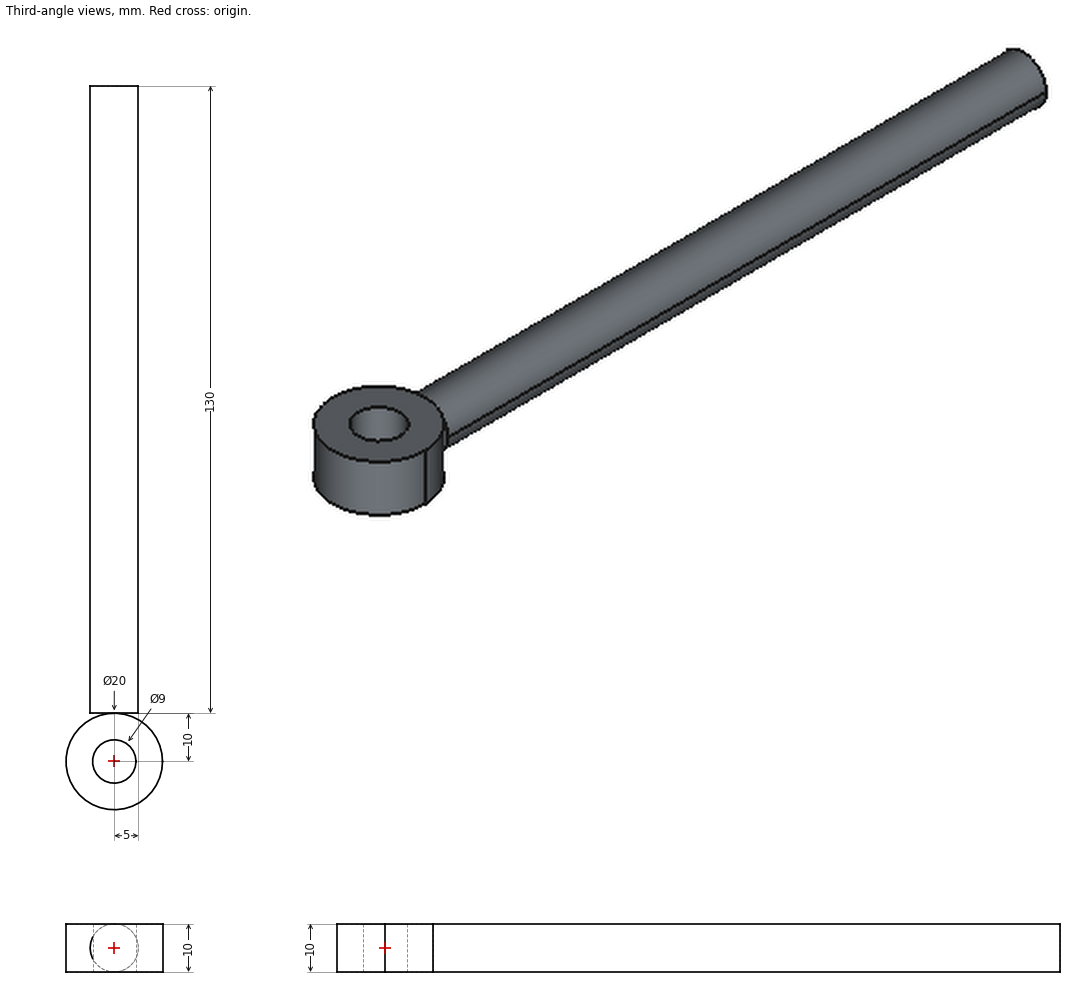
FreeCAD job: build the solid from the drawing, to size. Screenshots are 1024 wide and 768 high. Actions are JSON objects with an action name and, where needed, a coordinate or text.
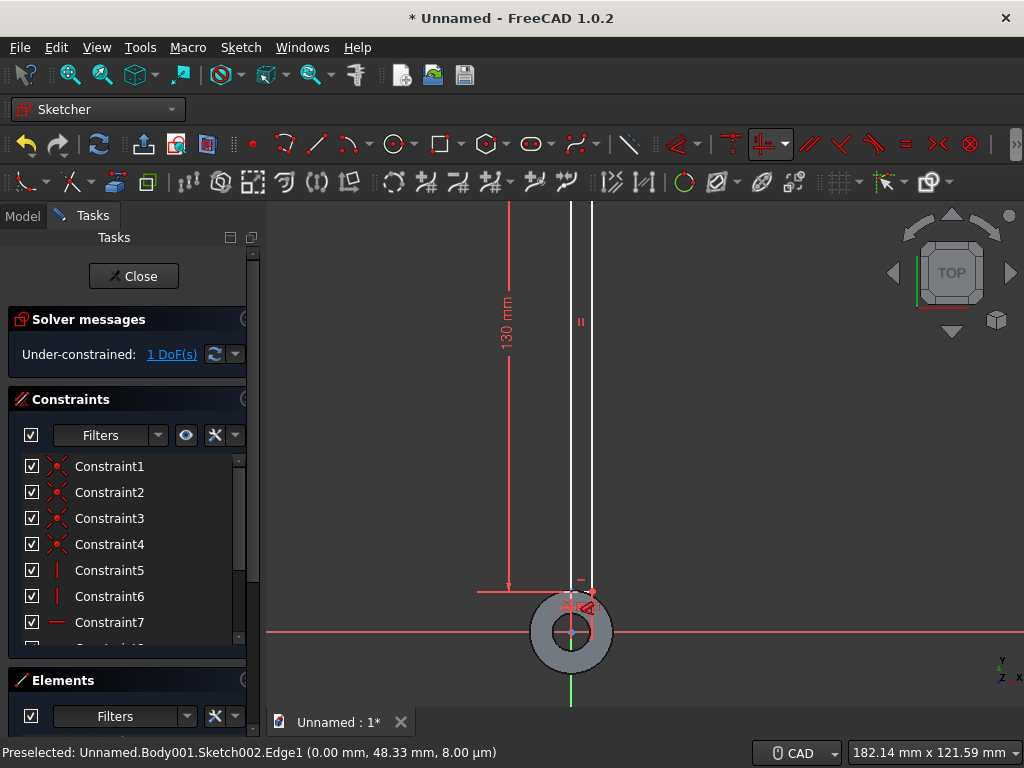
{"action": "left_click", "coordinate": [571, 592]}
{"action": "left_click", "coordinate": [489, 612]}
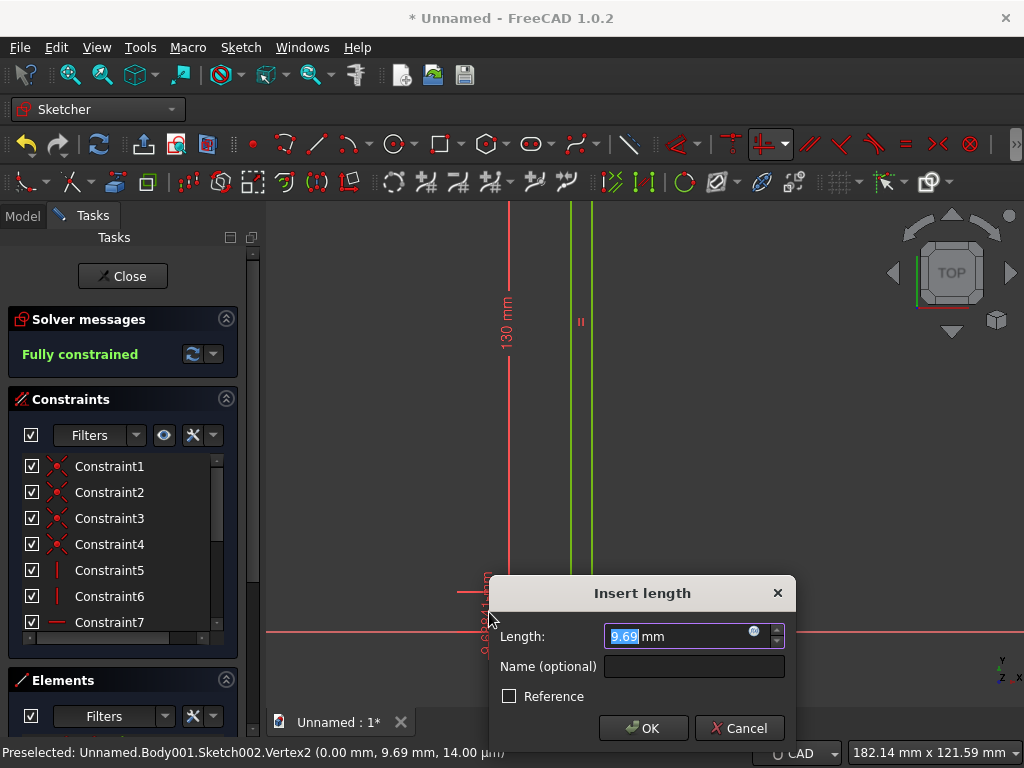
{"action": "type", "text": "10"}
{"action": "key", "text": "Return"}
{"action": "key", "text": "Escape"}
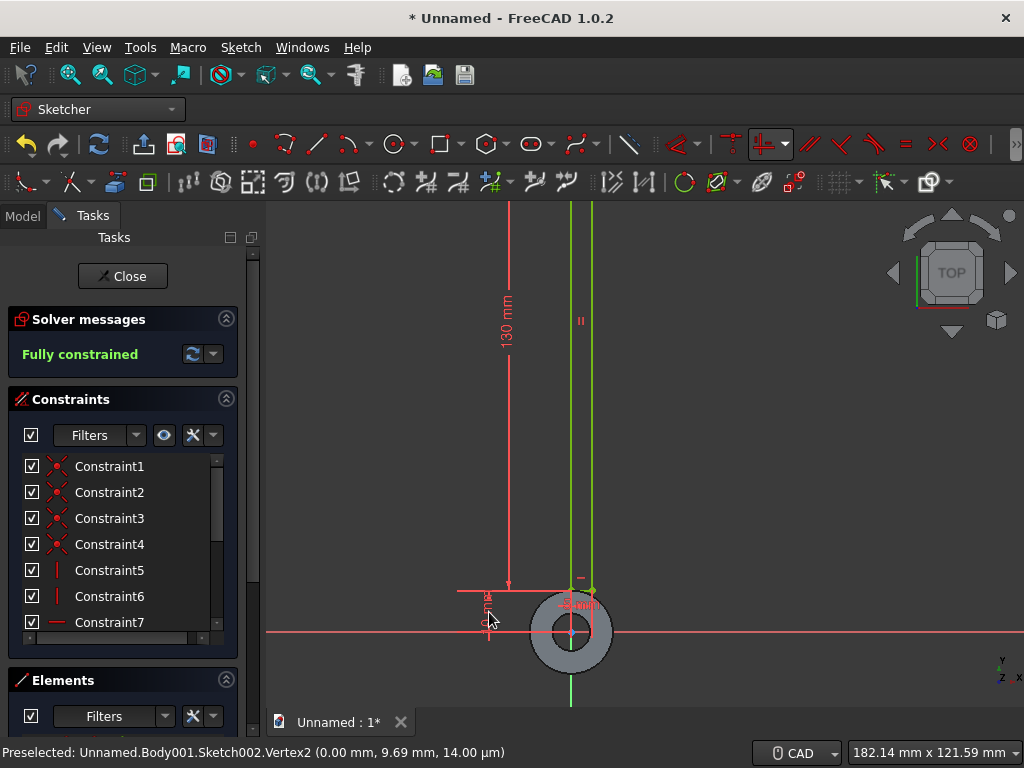
{"action": "left_click", "coordinate": [123, 276]}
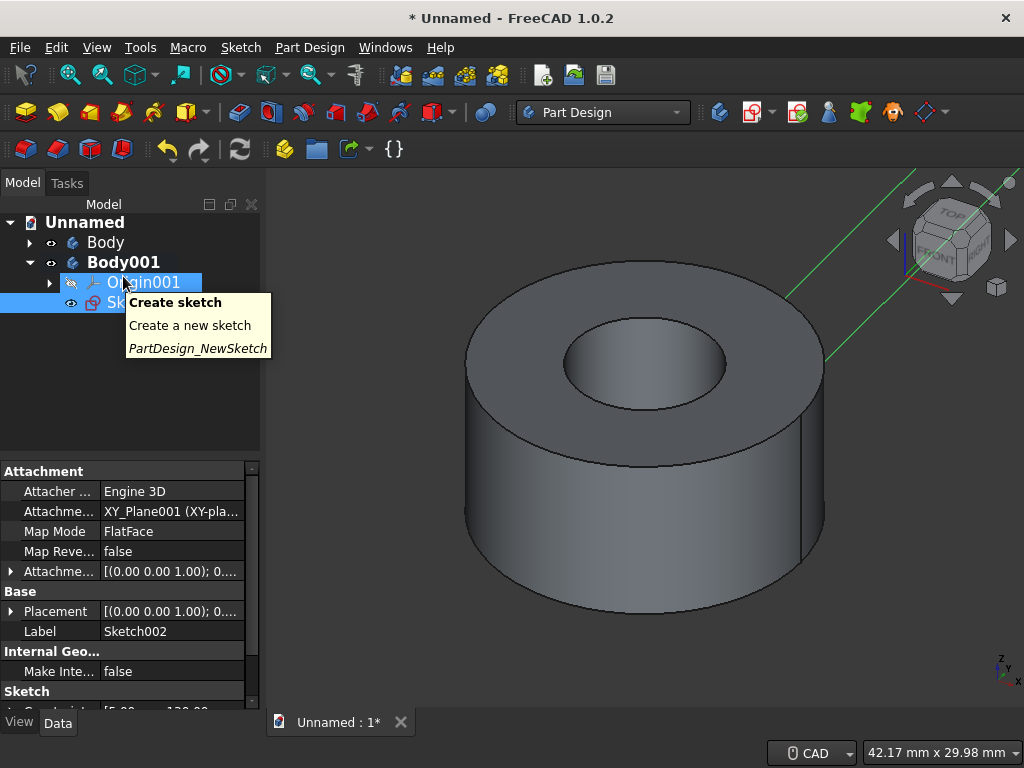
{"action": "left_click", "coordinate": [58, 112]}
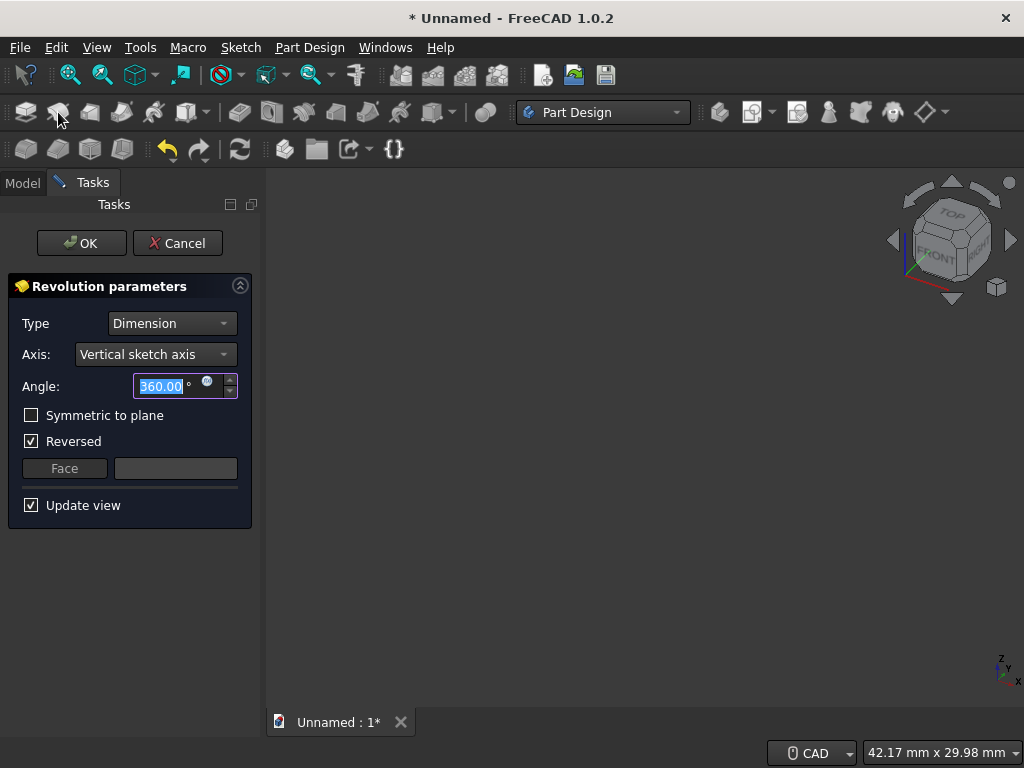
{"action": "left_click", "coordinate": [82, 243]}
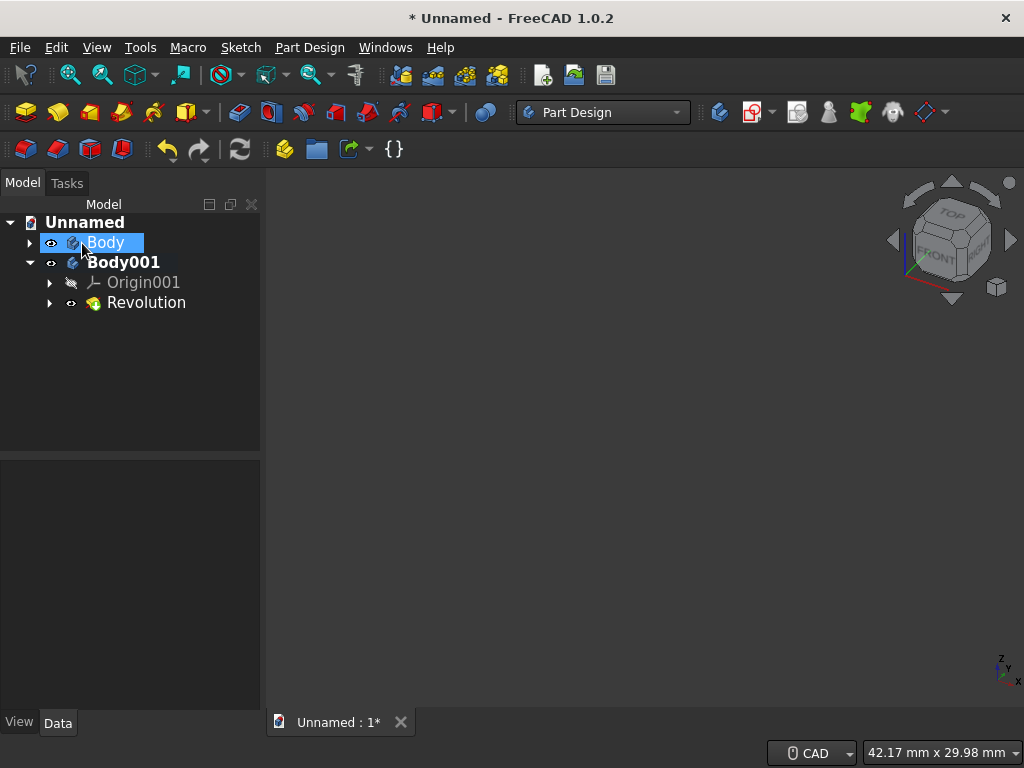
{"action": "key", "text": "0"}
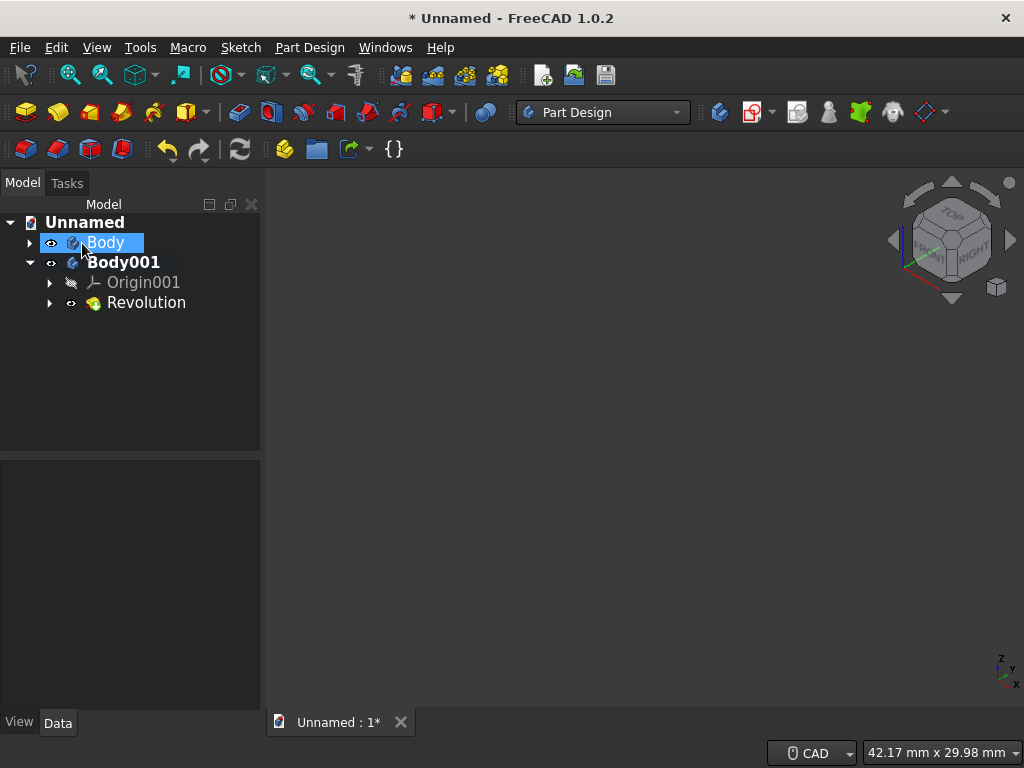
{"action": "left_click", "coordinate": [72, 76]}